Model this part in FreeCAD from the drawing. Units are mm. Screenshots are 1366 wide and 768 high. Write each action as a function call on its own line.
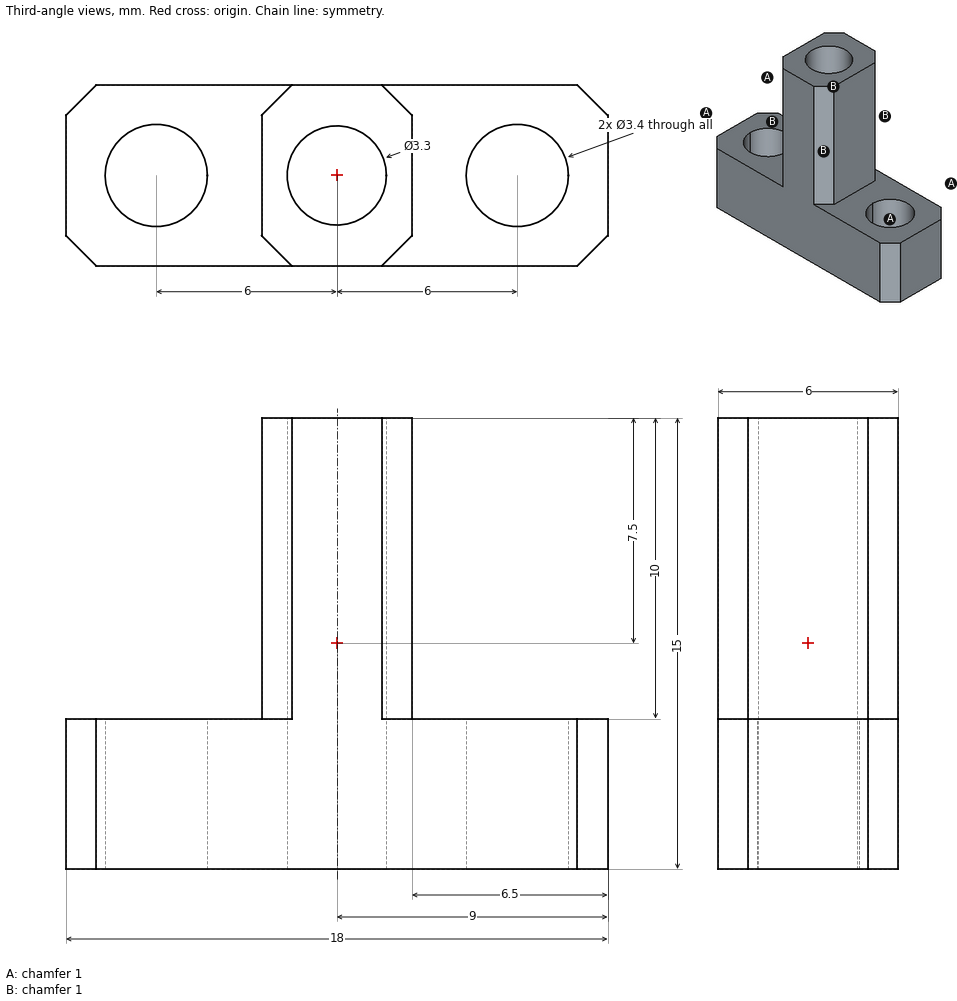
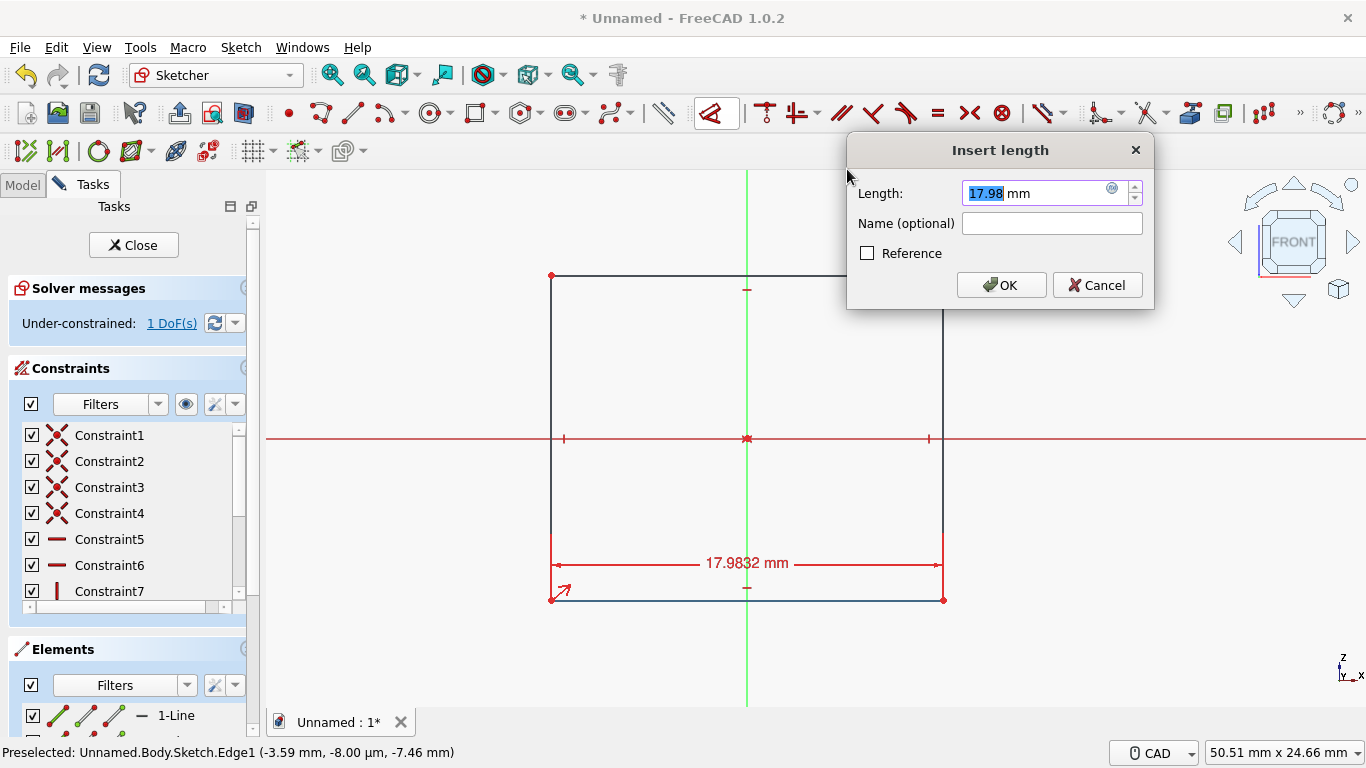
text(18)
key(Return)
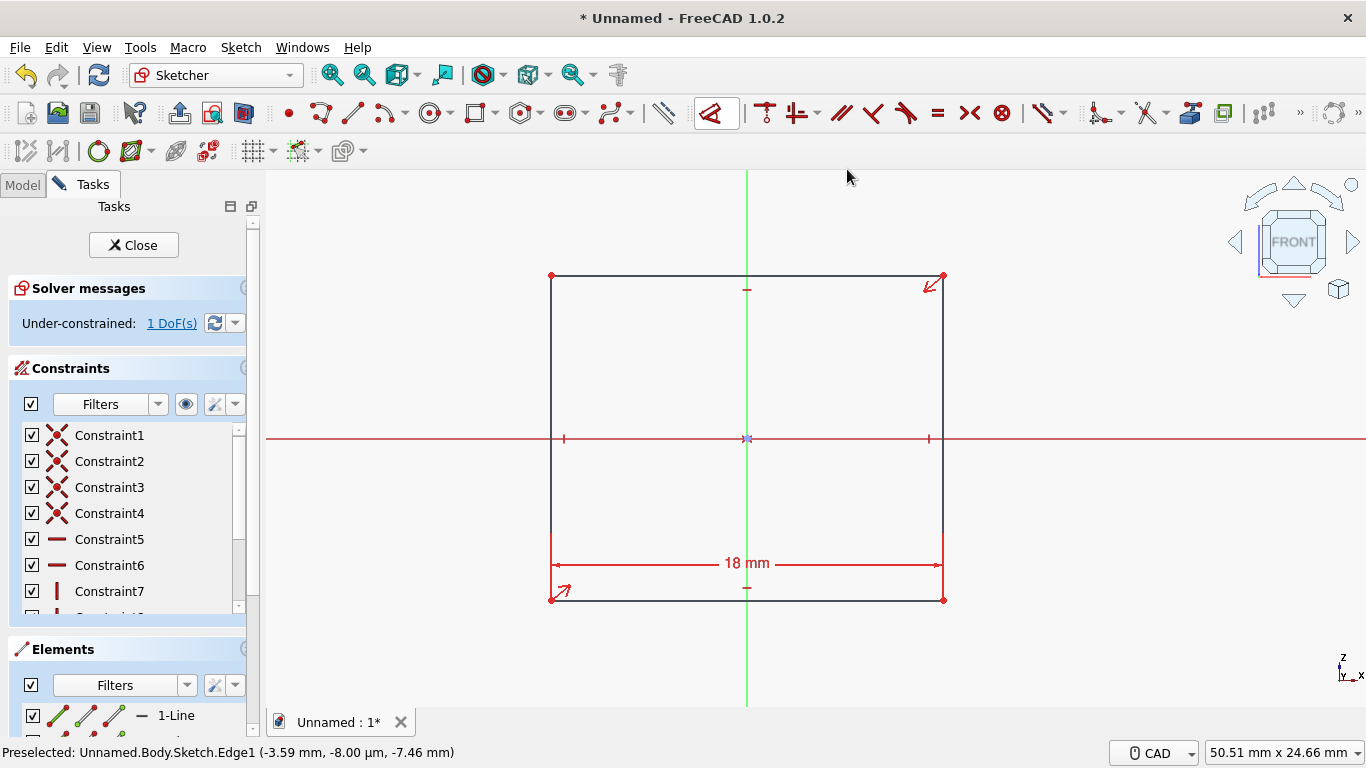
click(943, 503)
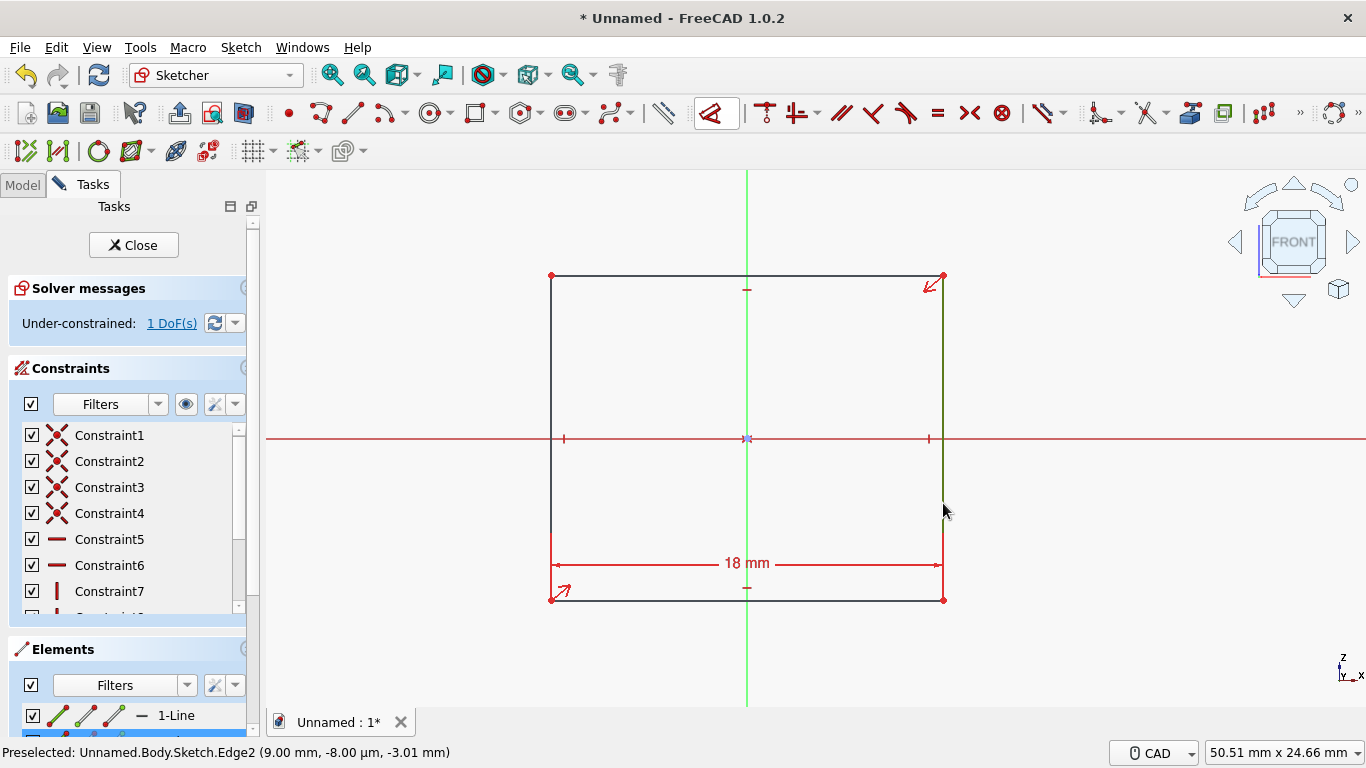
key(i)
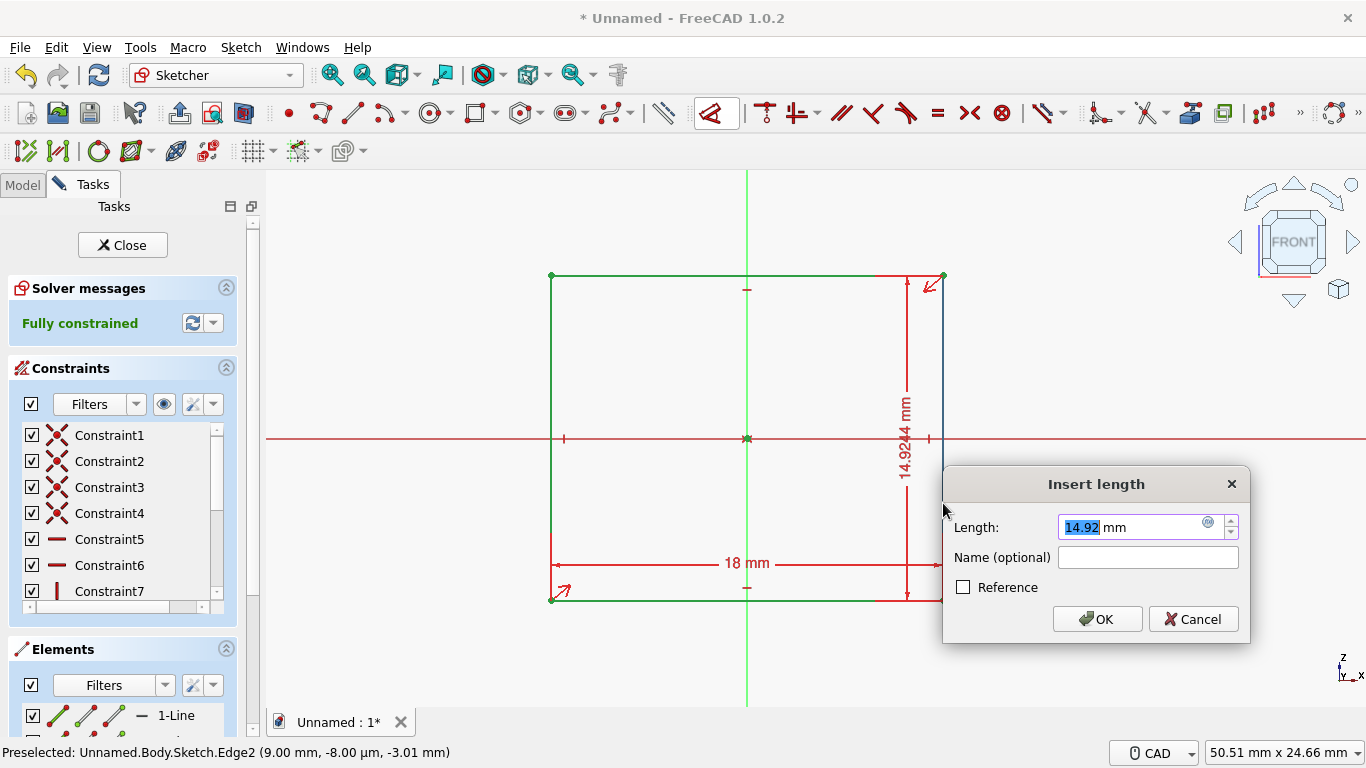
text(15)
key(Return)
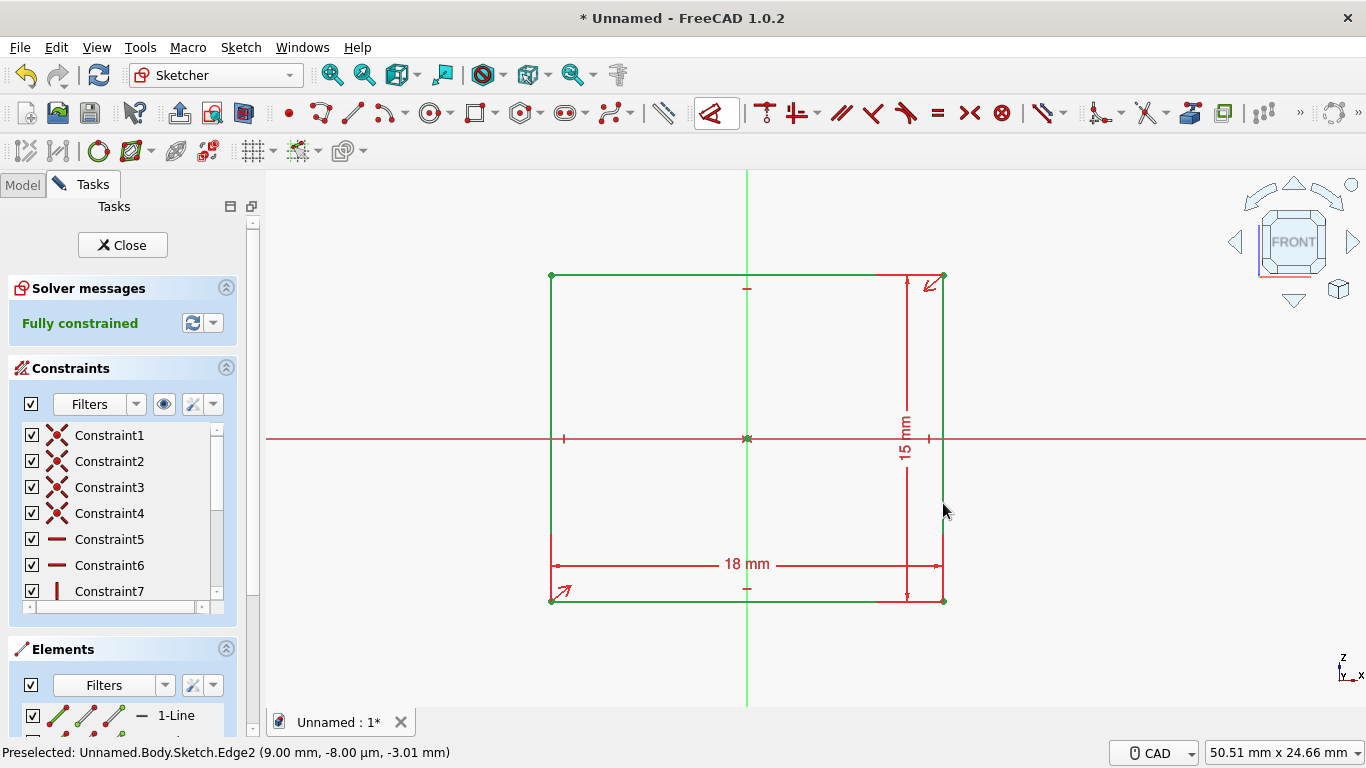
click(123, 245)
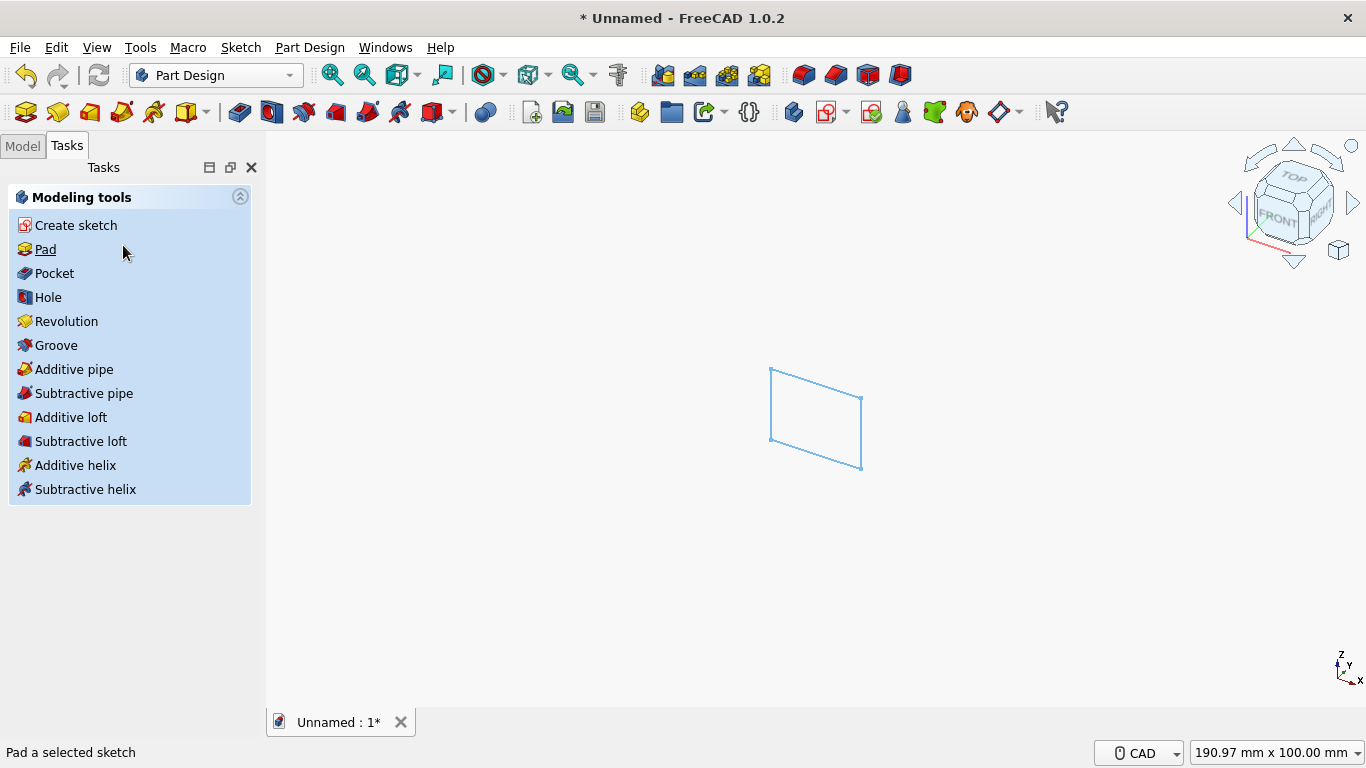
click(26, 112)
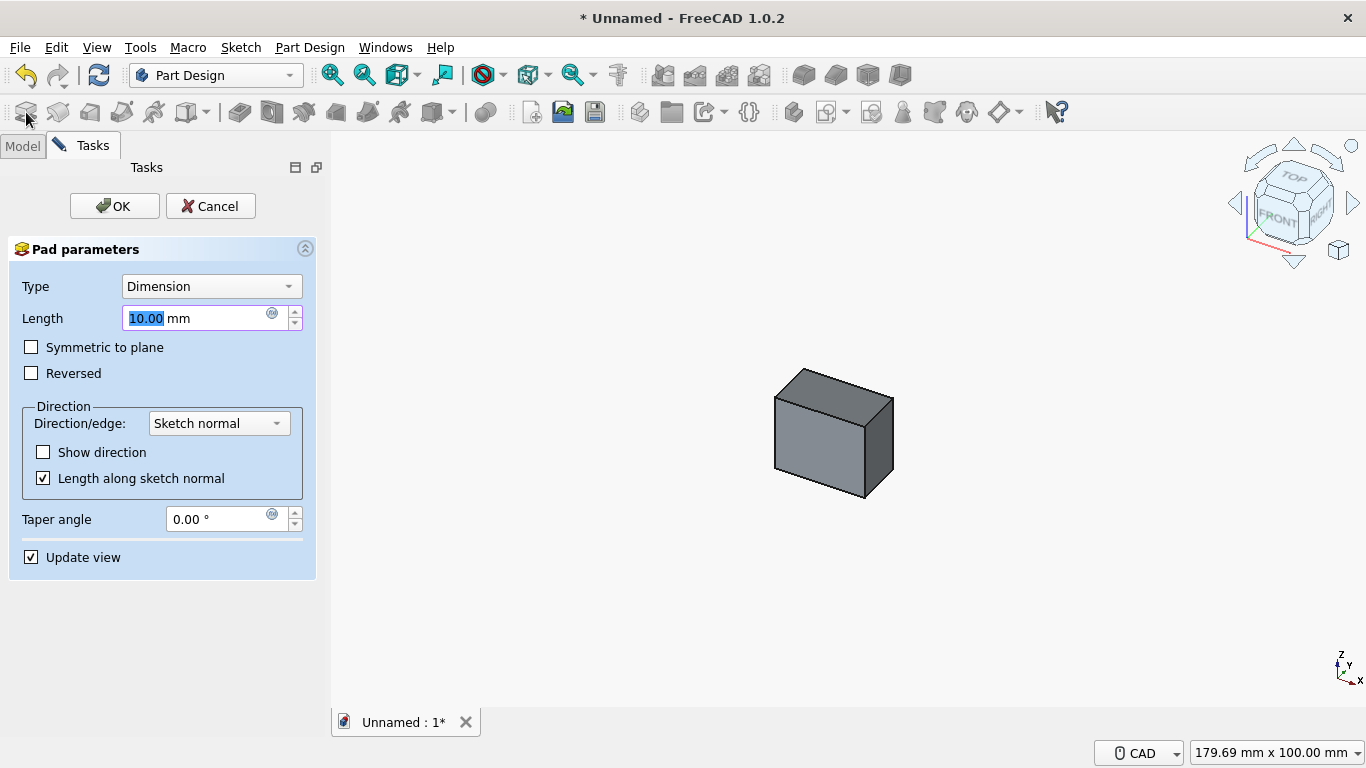
text(6)
key(Tab)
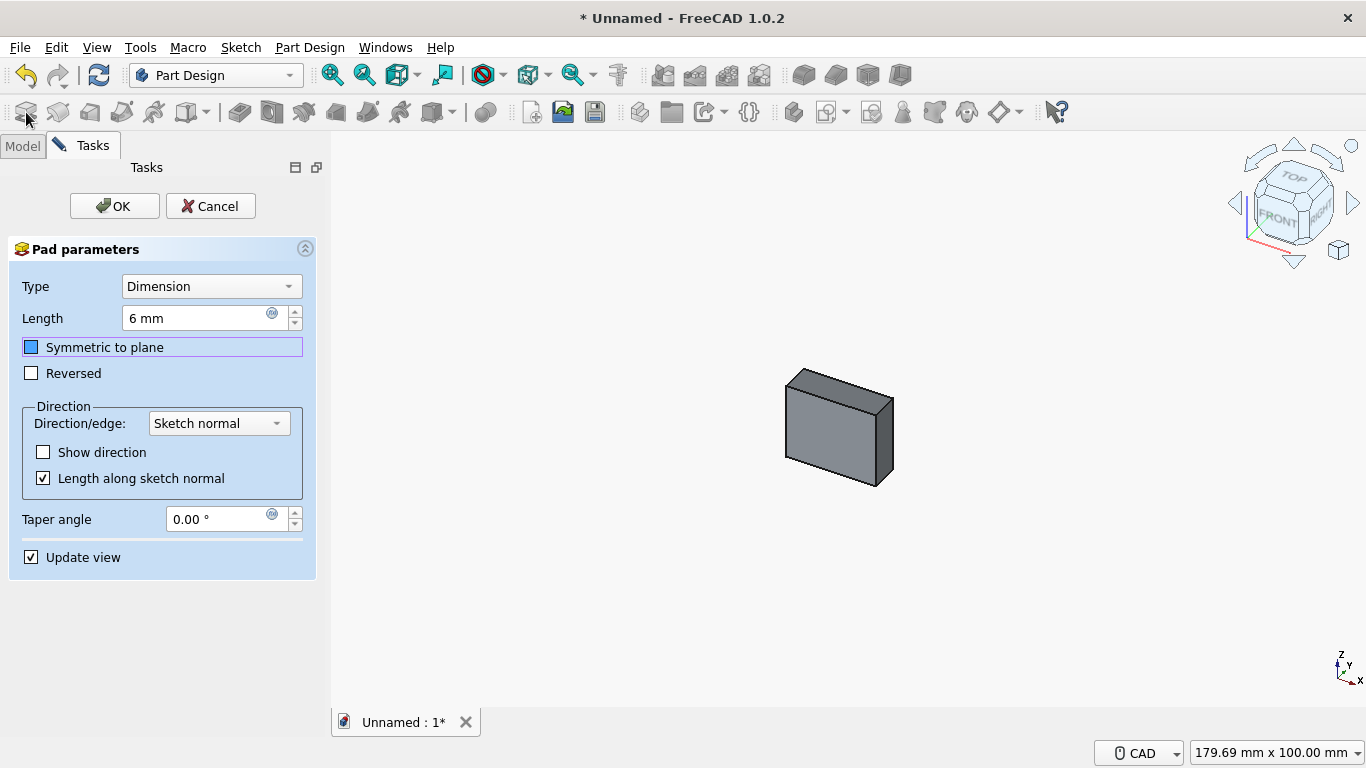
click(30, 347)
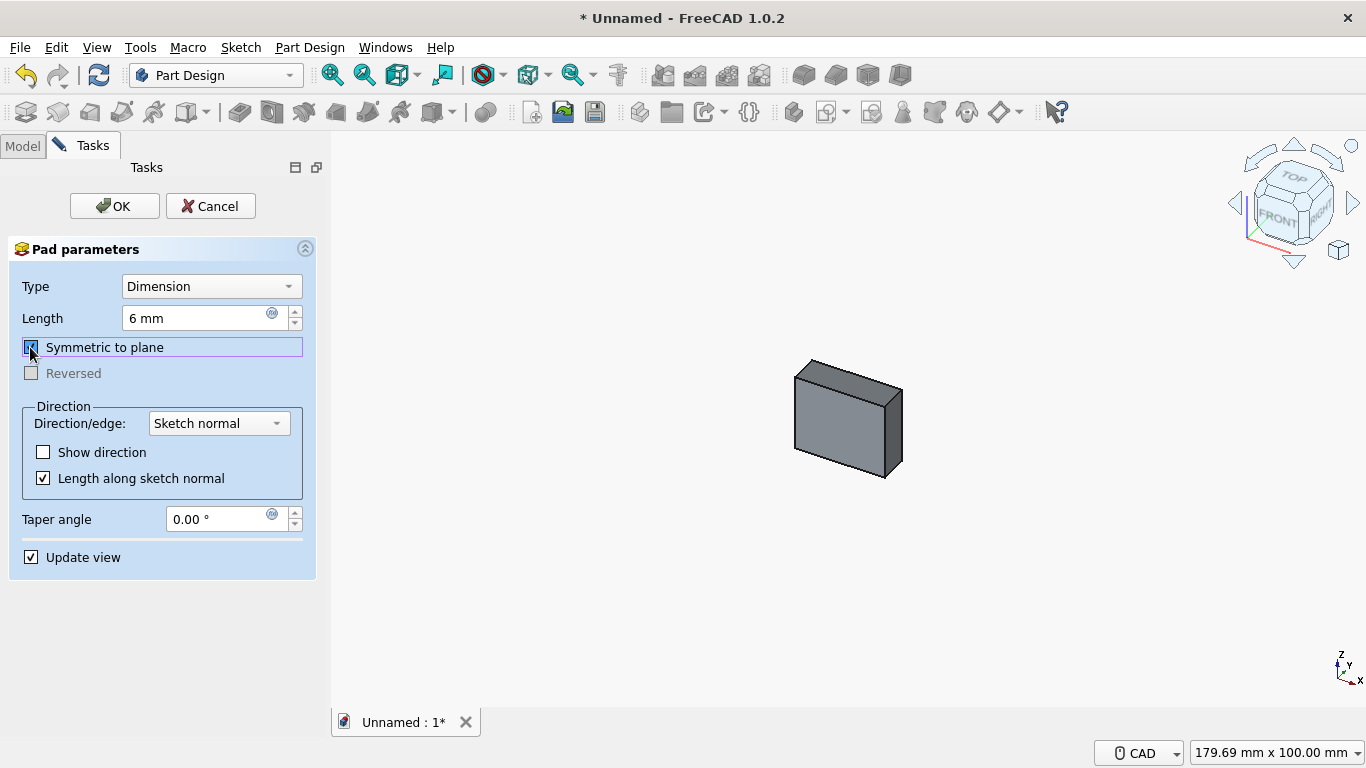
click(115, 206)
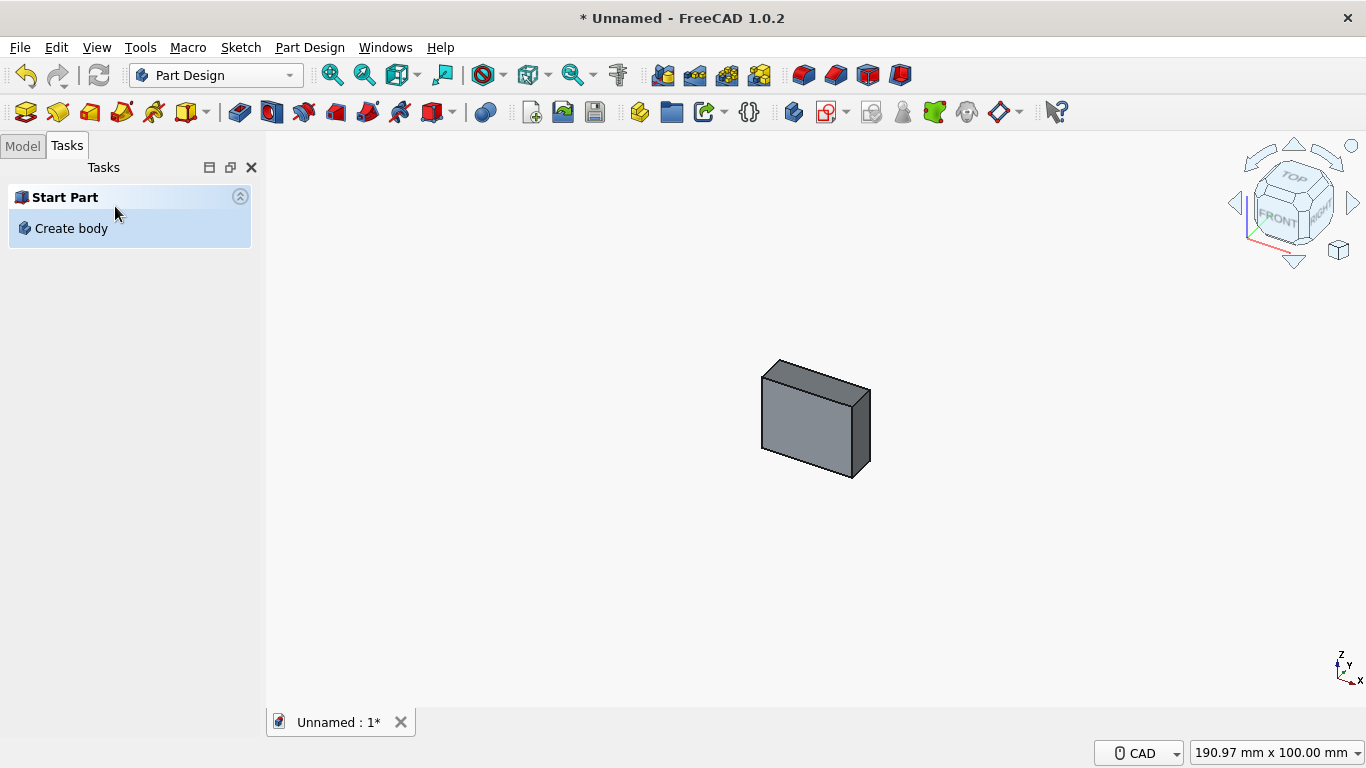
click(334, 76)